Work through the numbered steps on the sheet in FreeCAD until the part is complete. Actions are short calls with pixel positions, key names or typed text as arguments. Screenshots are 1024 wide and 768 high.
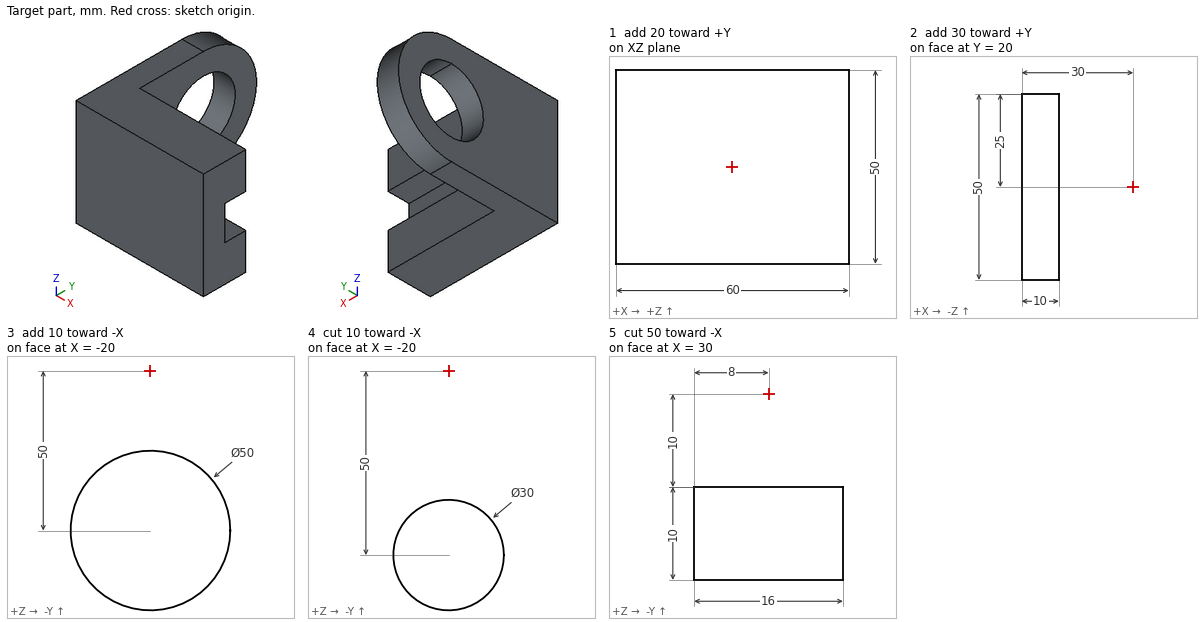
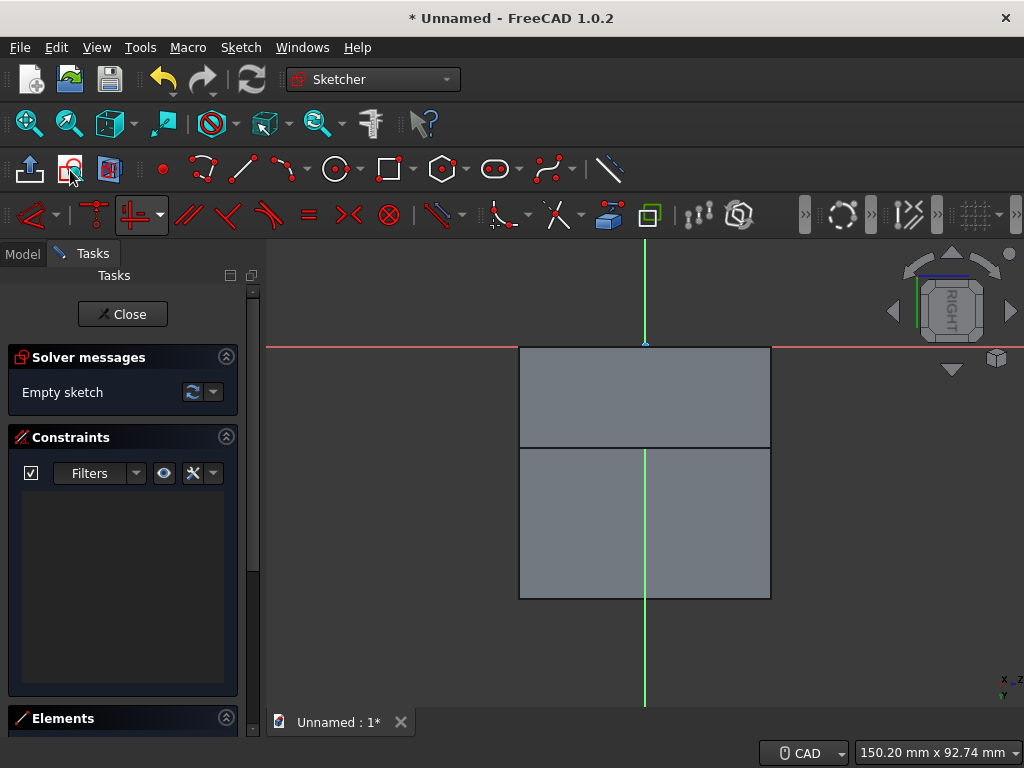
scroll(294, 267, down, 1)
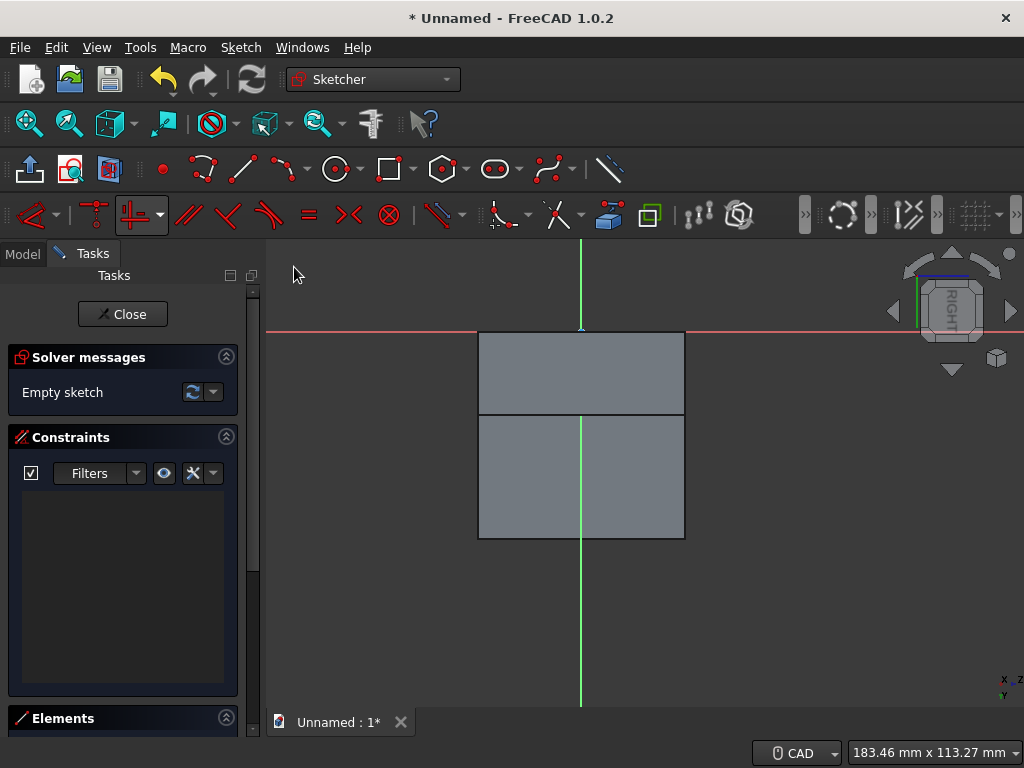
click(336, 170)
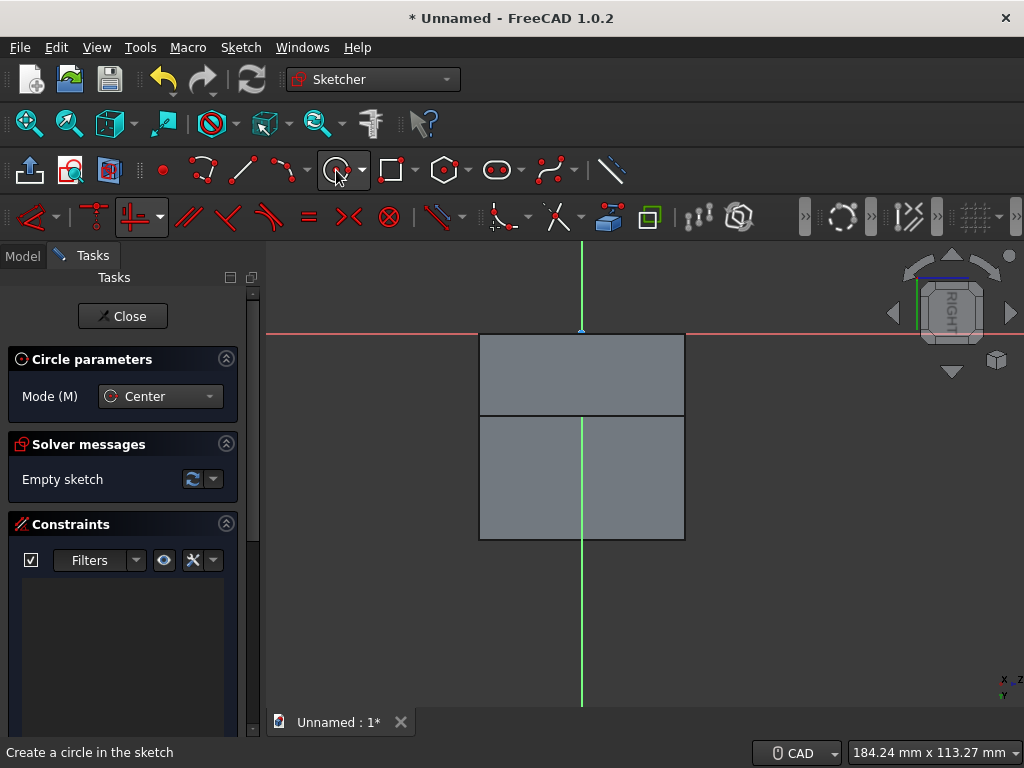
click(582, 540)
click(654, 467)
key(Escape)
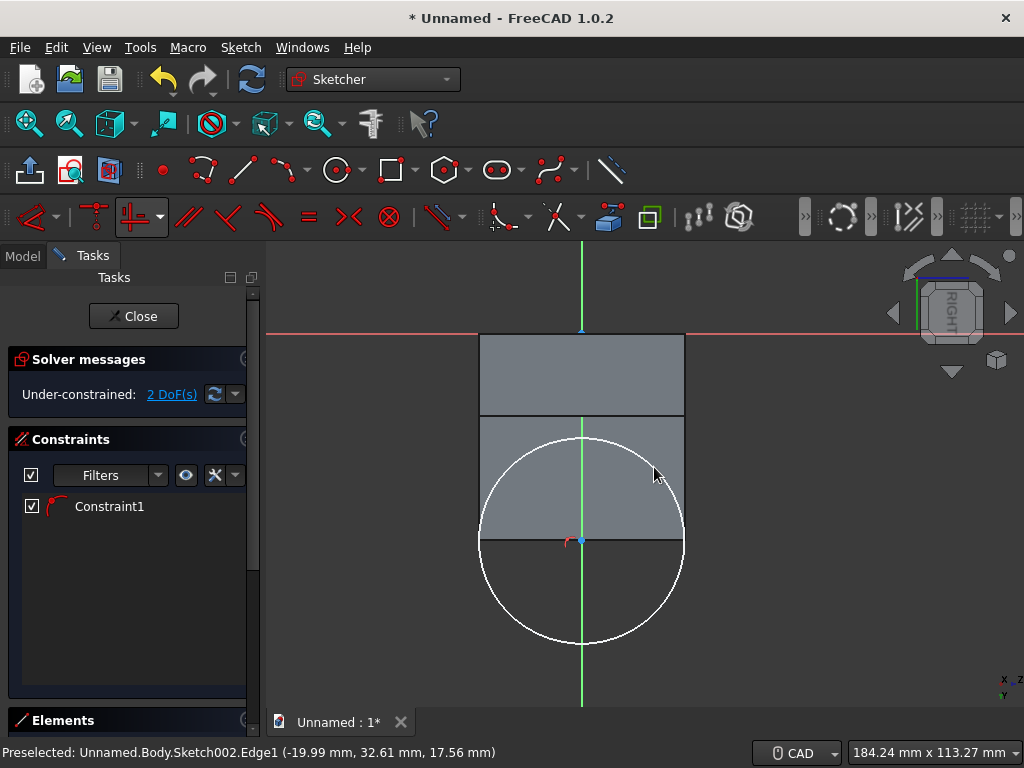
click(32, 218)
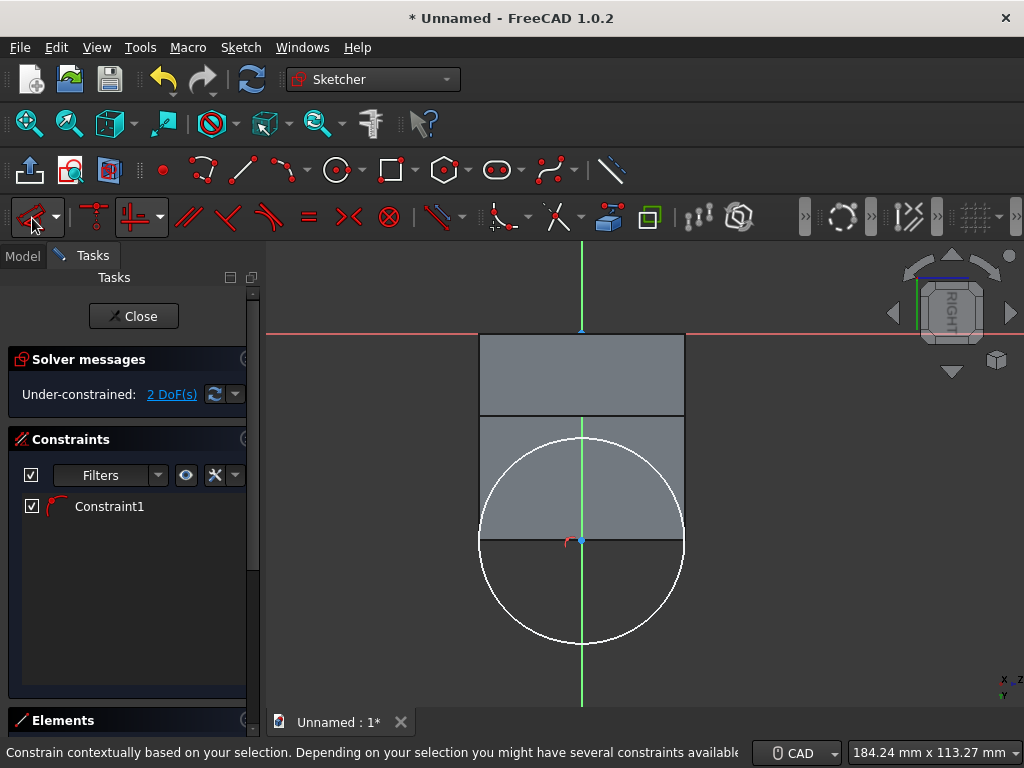
click(654, 468)
click(677, 445)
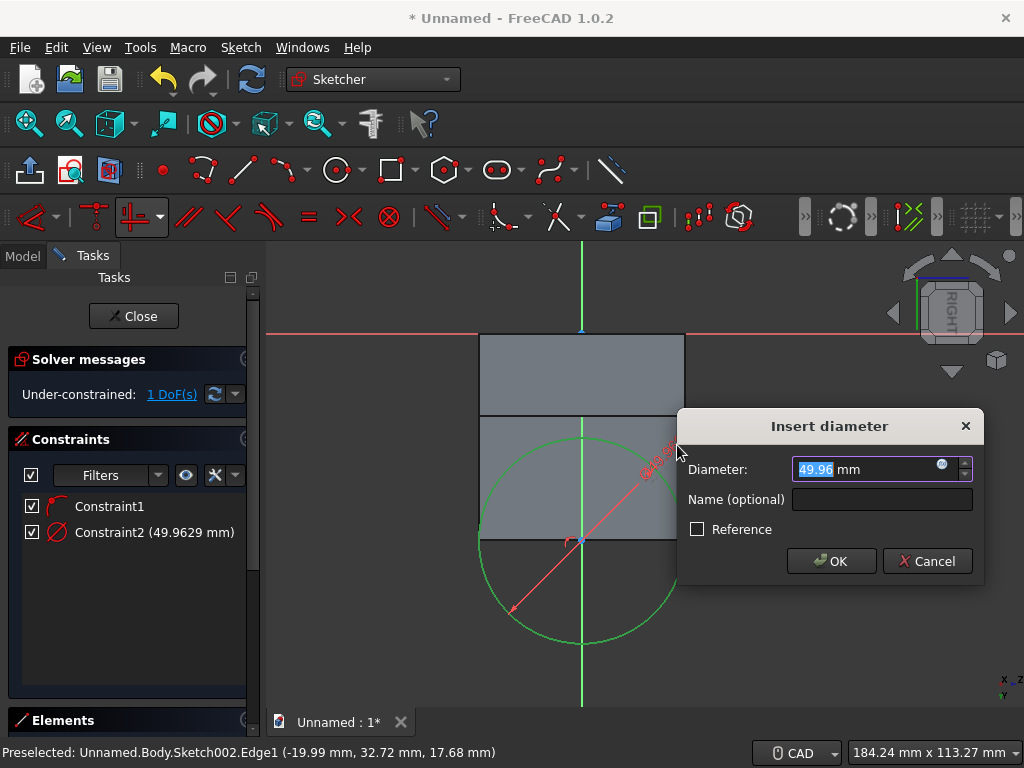
text(50)
key(Return)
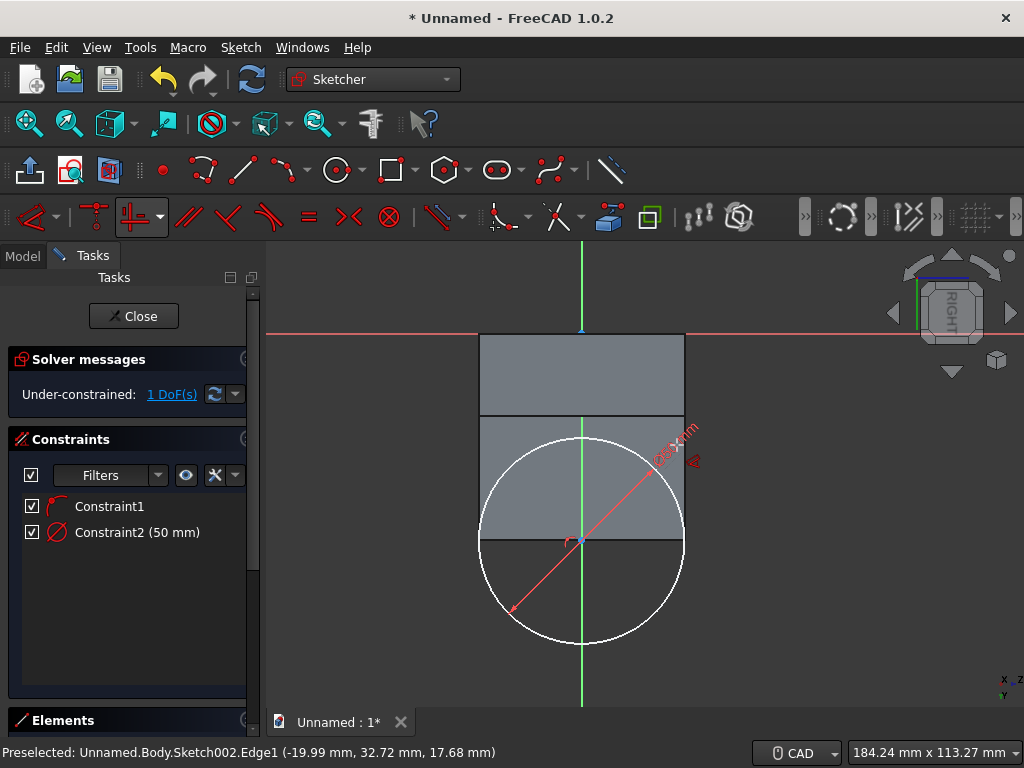
click(582, 541)
click(616, 390)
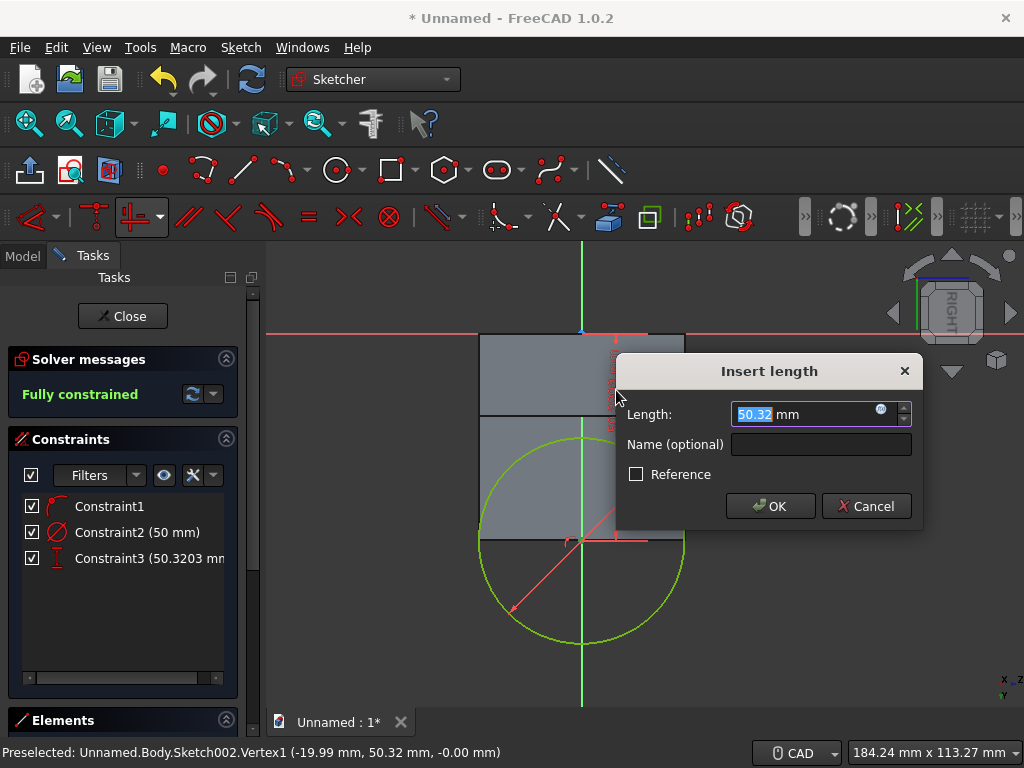
text(50)
key(Return)
key(Escape)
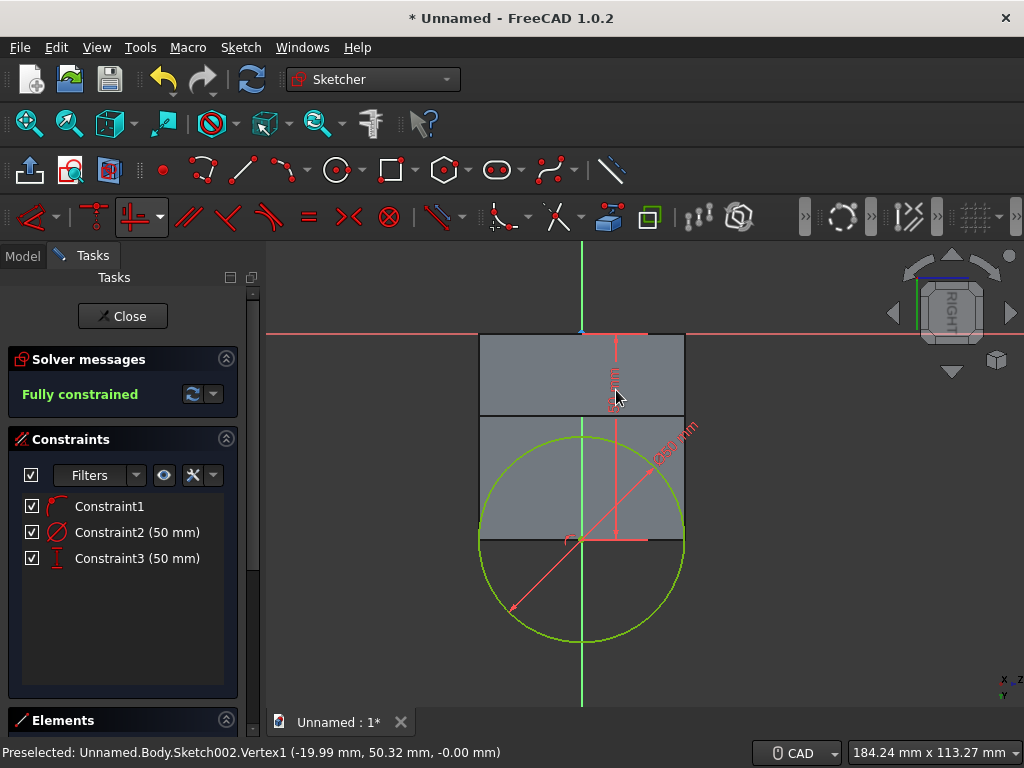
click(123, 316)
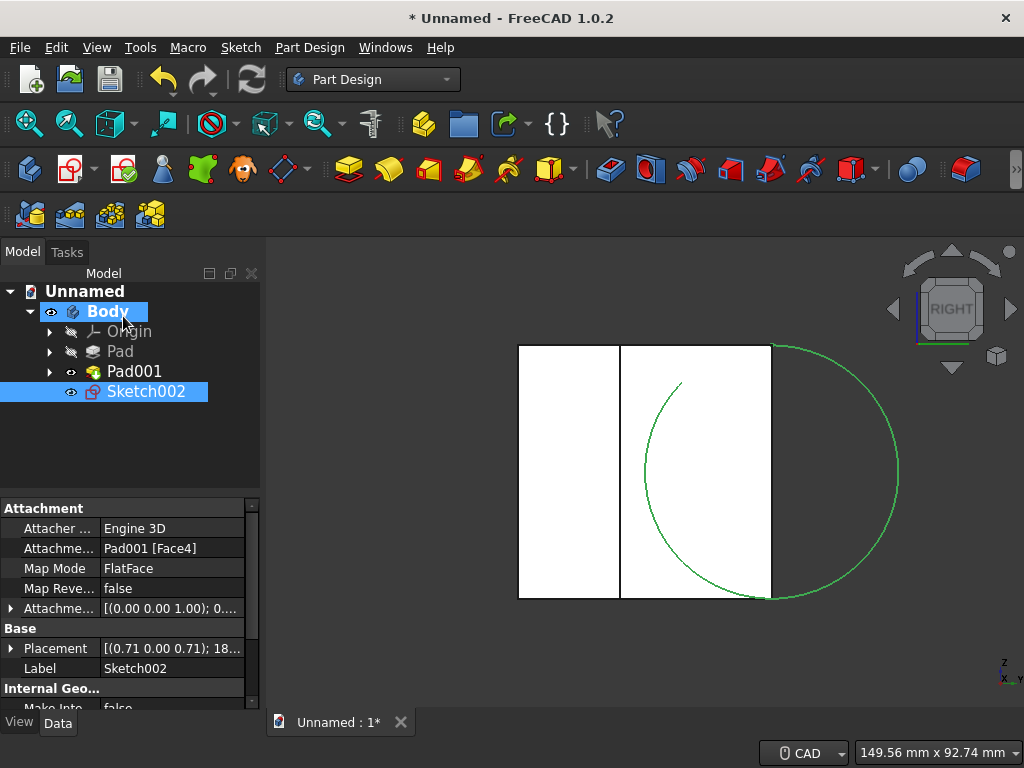
click(350, 170)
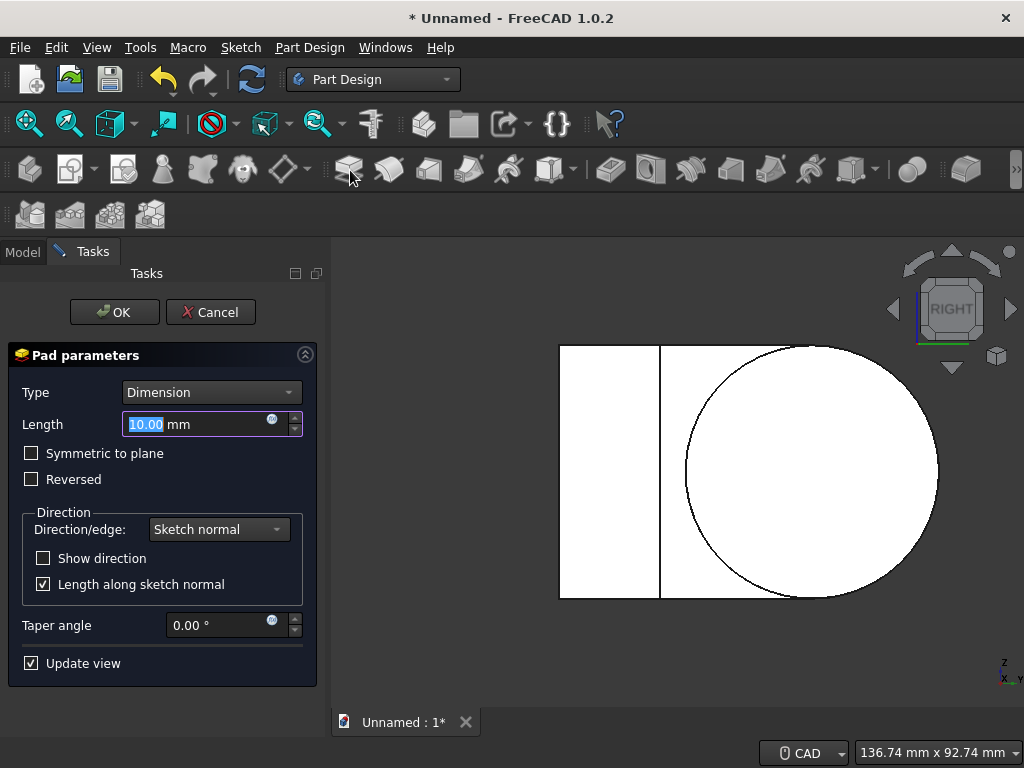
text(10)
key(Tab)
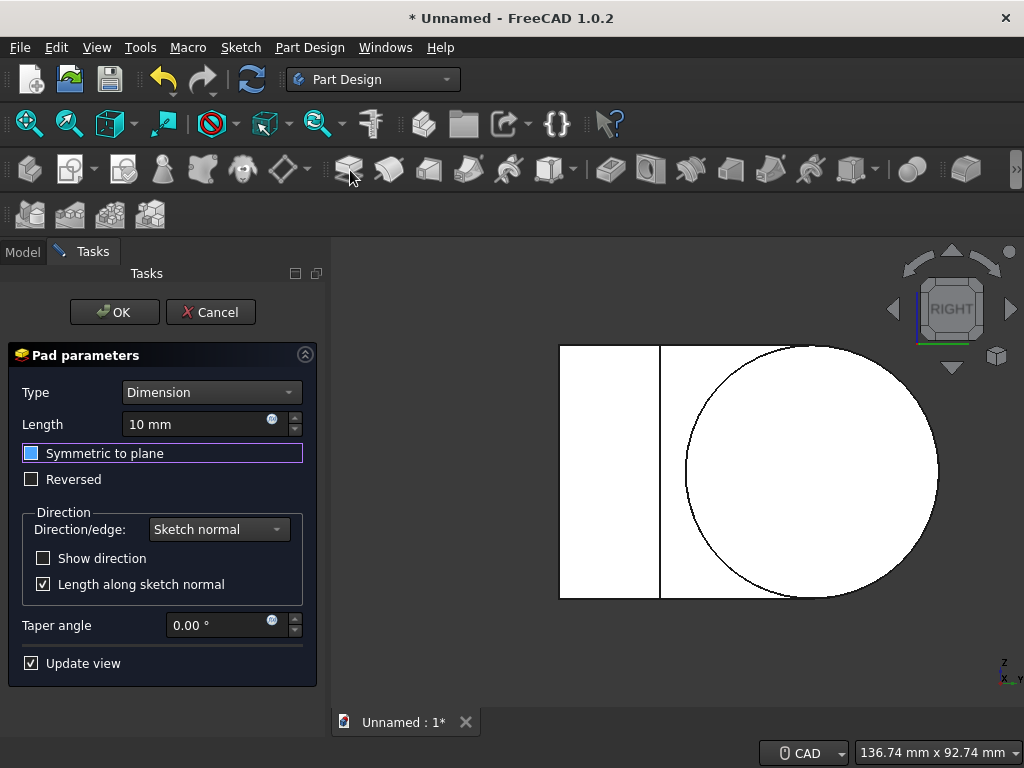
click(30, 479)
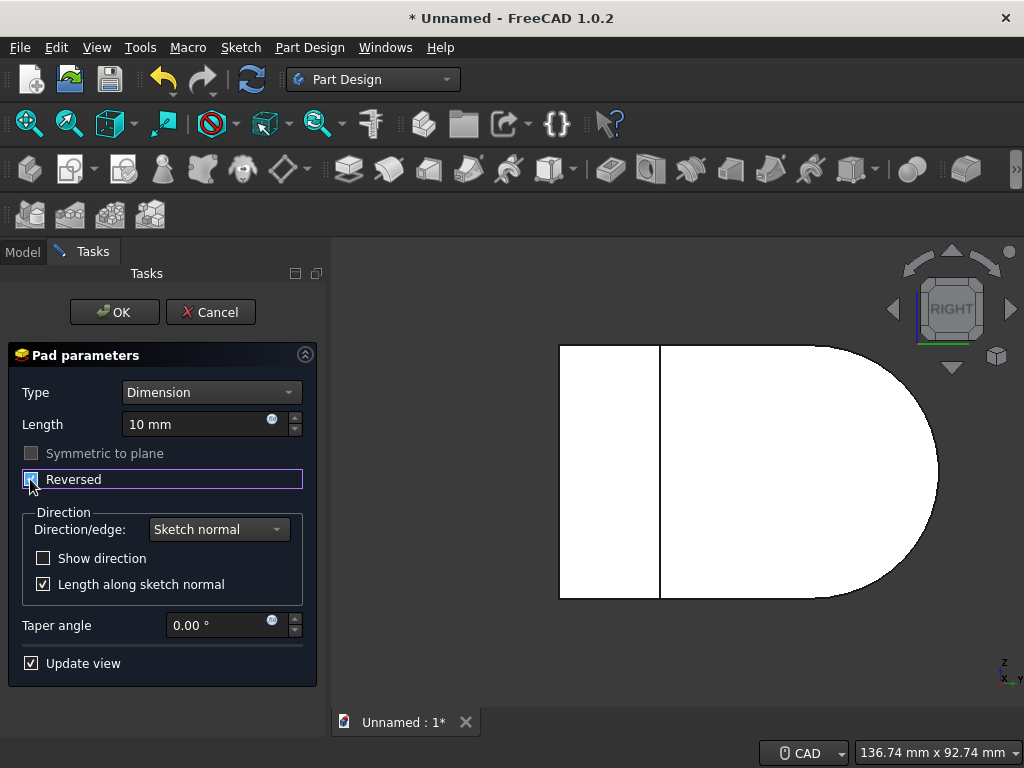
click(115, 312)